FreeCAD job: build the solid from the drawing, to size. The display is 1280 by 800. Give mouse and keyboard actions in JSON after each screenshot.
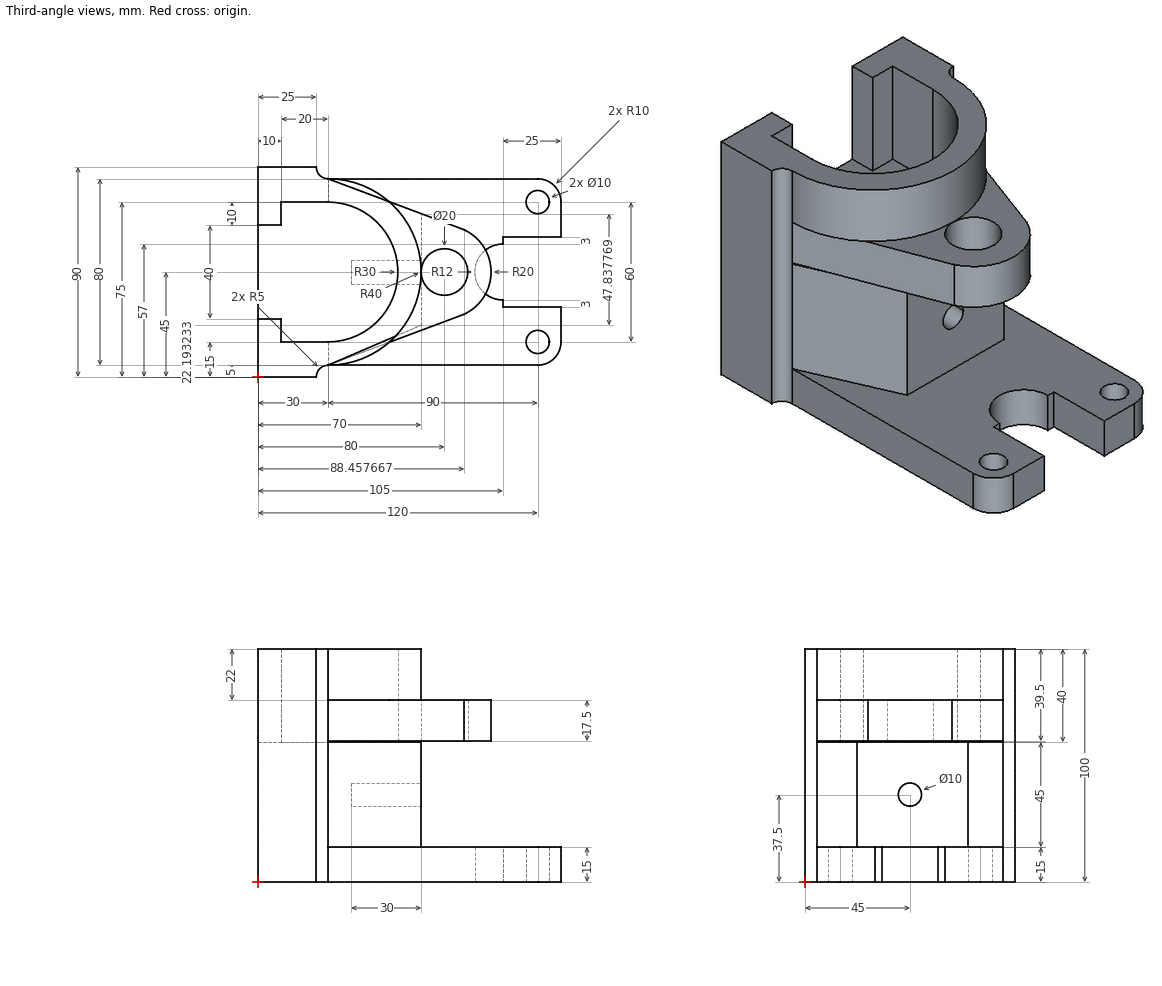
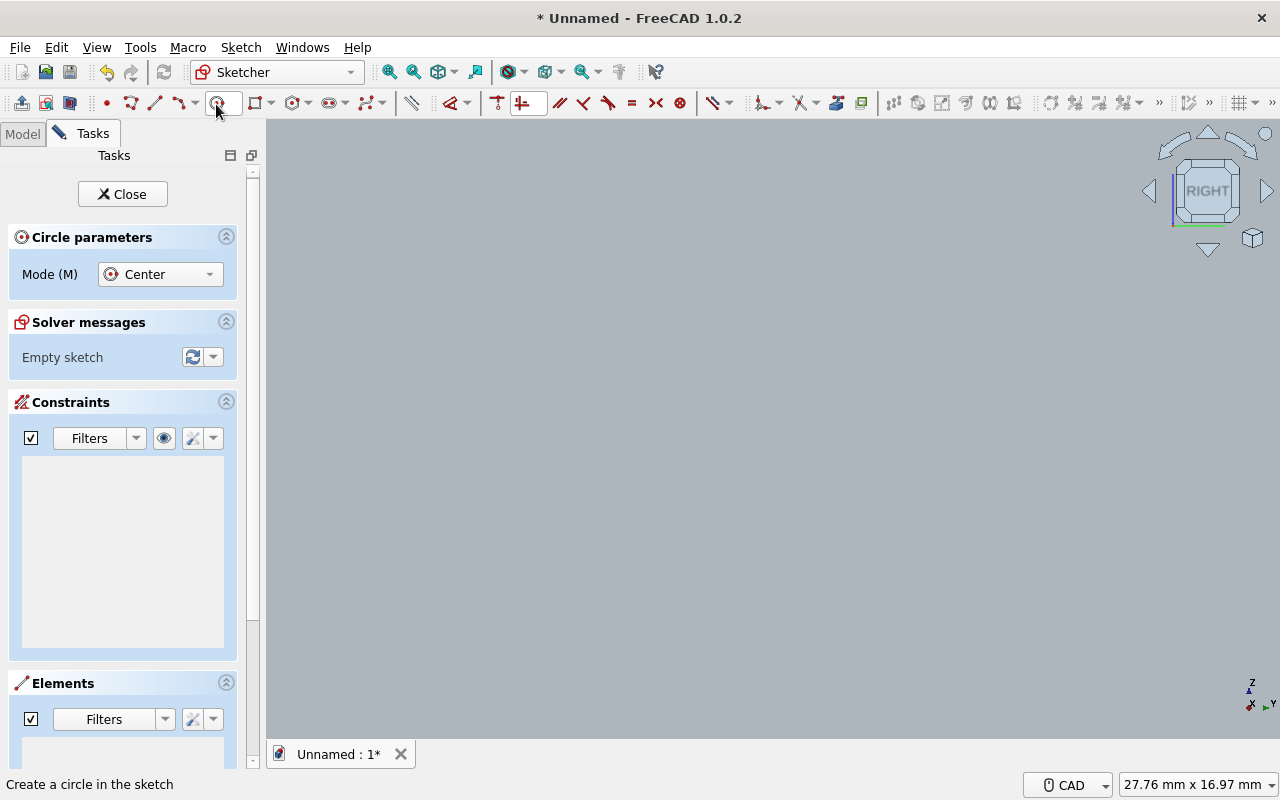
{"action": "left_click", "coordinate": [698, 419]}
{"action": "left_click", "coordinate": [827, 290]}
{"action": "key", "text": "Escape"}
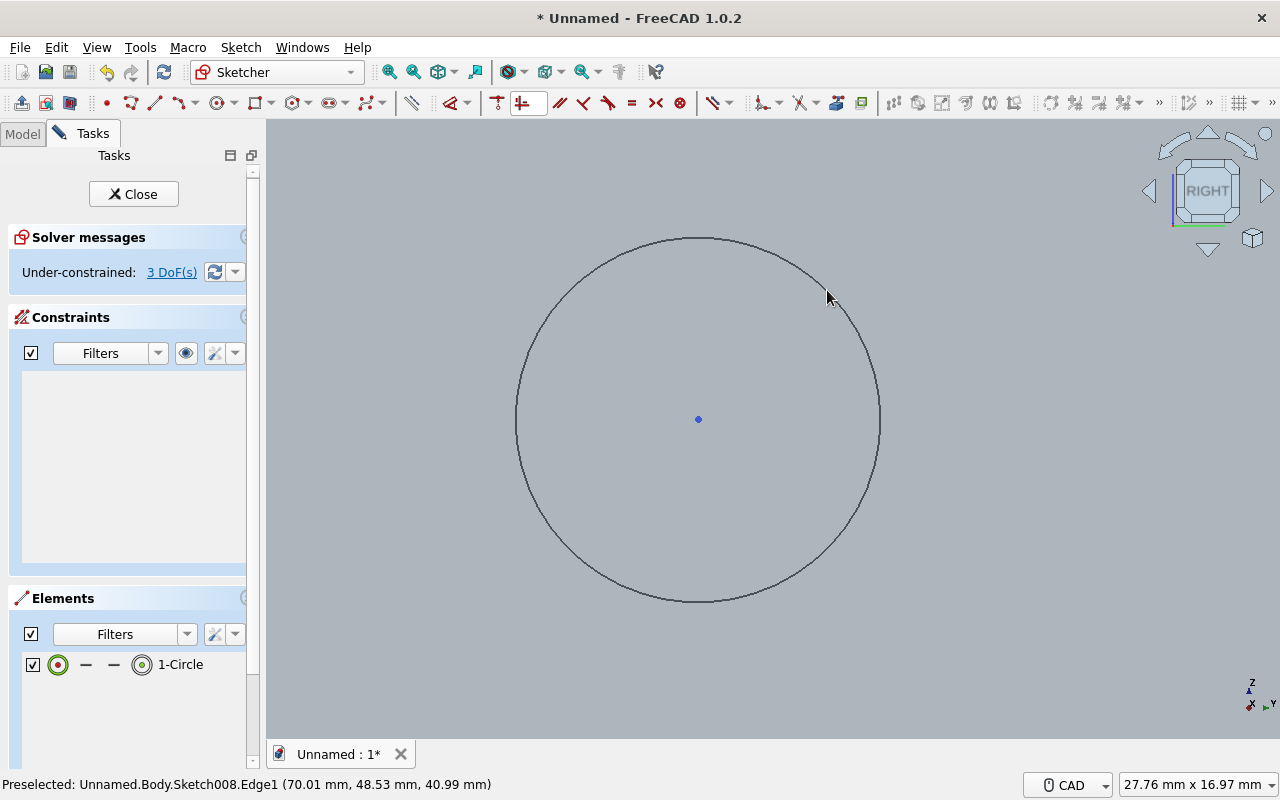
{"action": "left_click", "coordinate": [450, 104]}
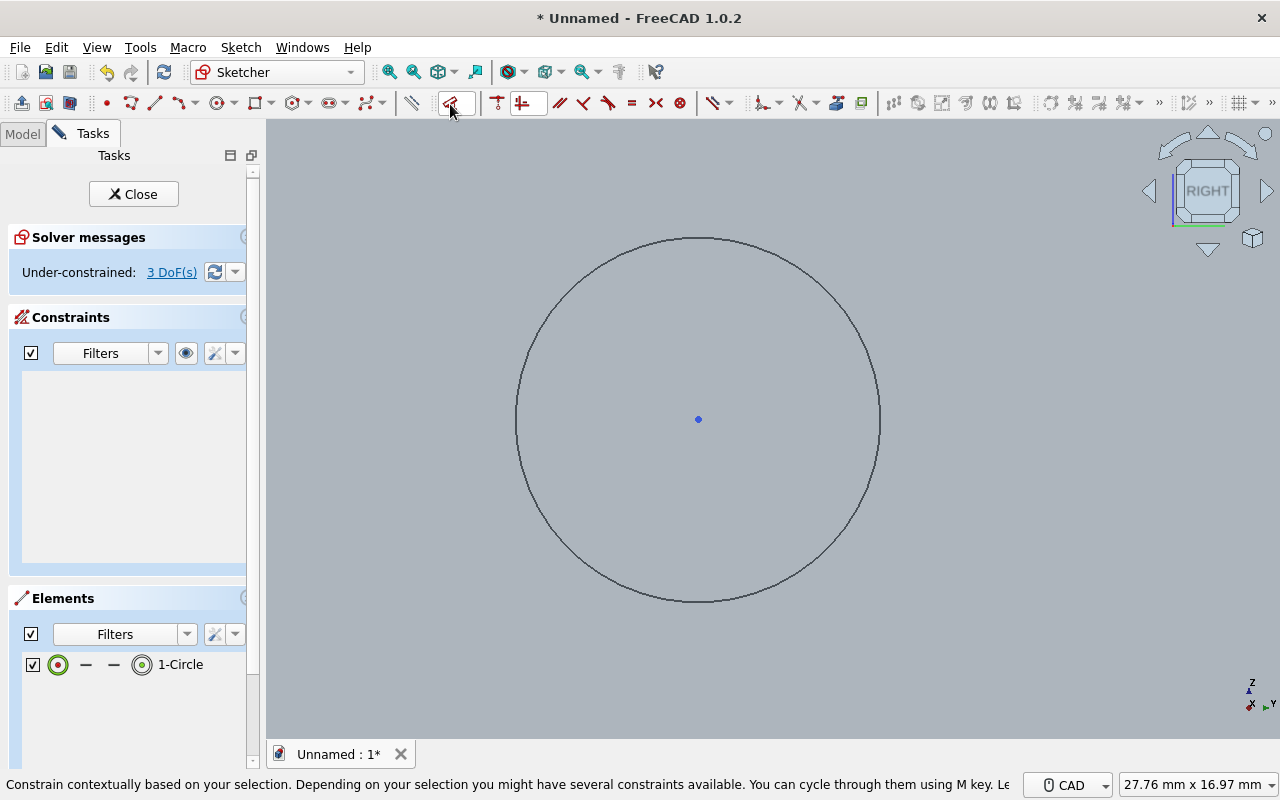
{"action": "left_click", "coordinate": [827, 291]}
{"action": "left_click", "coordinate": [850, 268]}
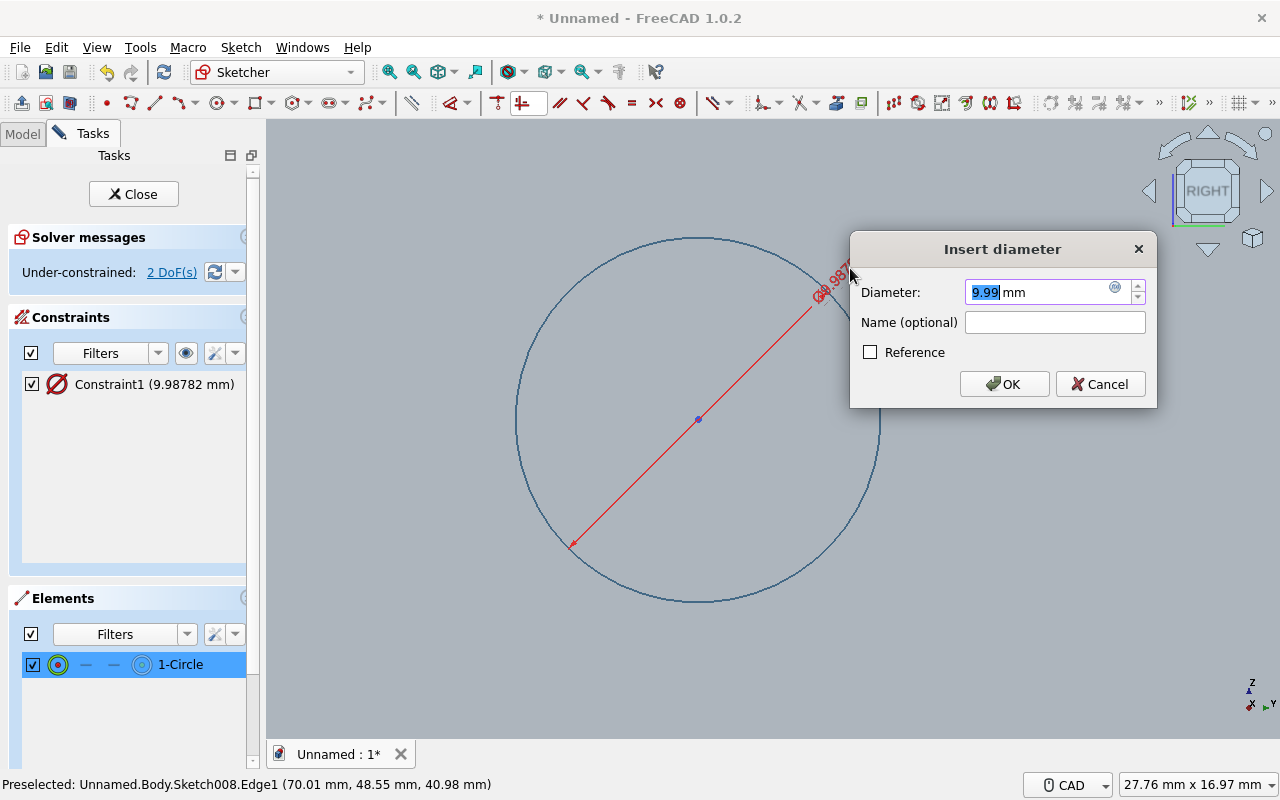
{"action": "type", "text": "10"}
{"action": "key", "text": "Return"}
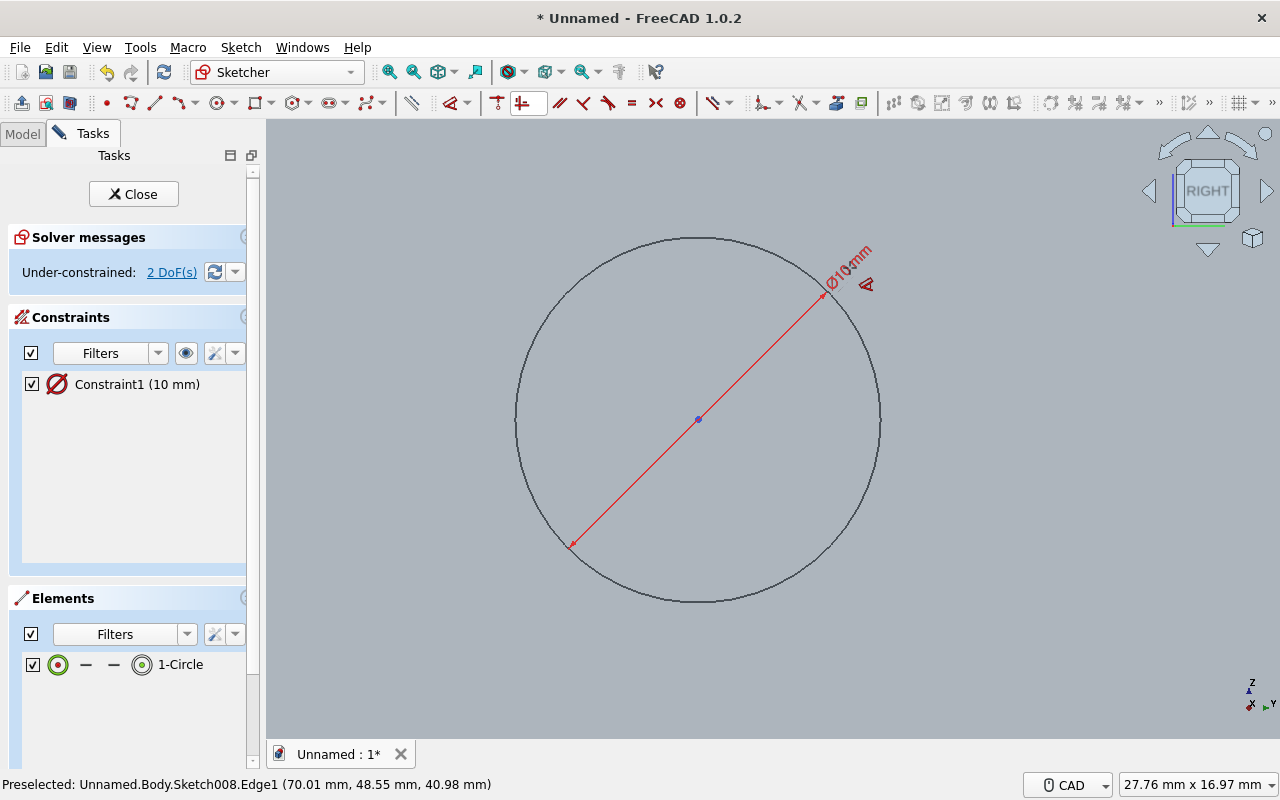
{"action": "left_click", "coordinate": [698, 420]}
{"action": "left_click", "coordinate": [496, 386]}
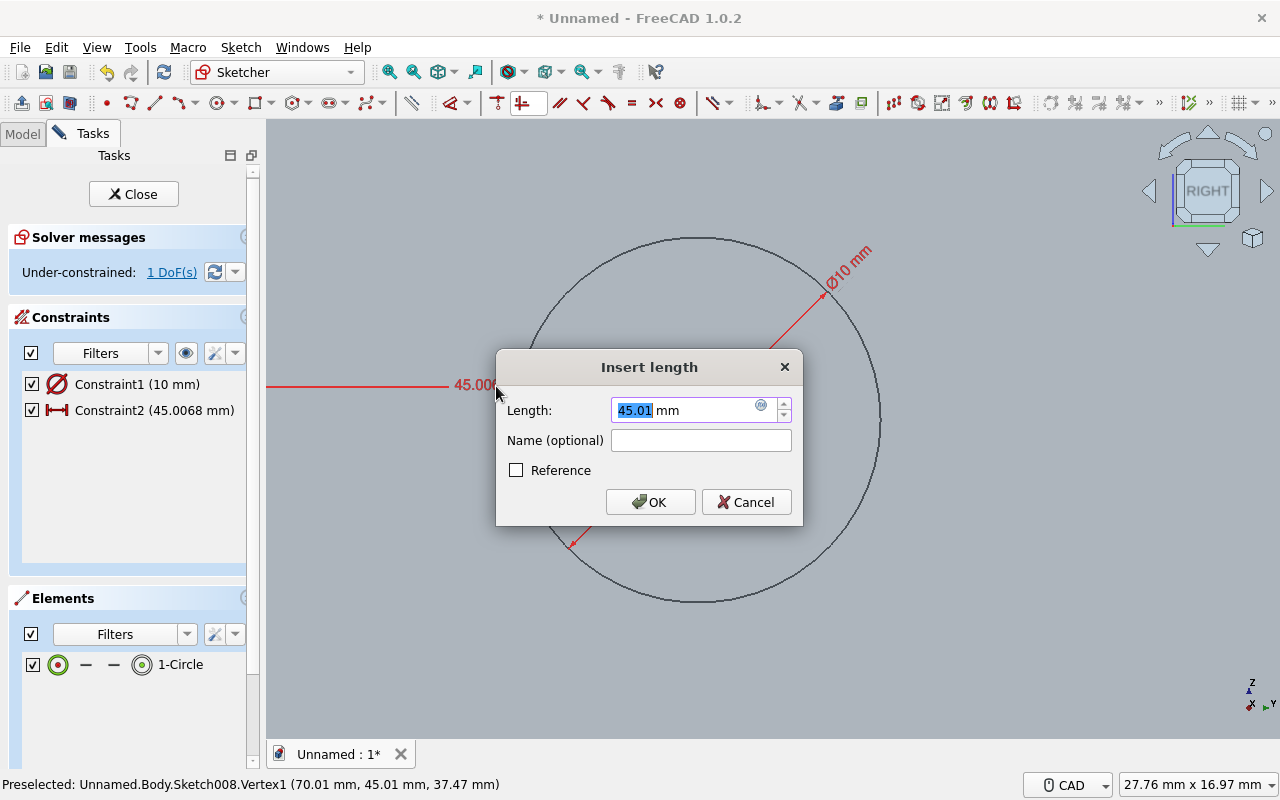
{"action": "type", "text": "45"}
{"action": "key", "text": "Return"}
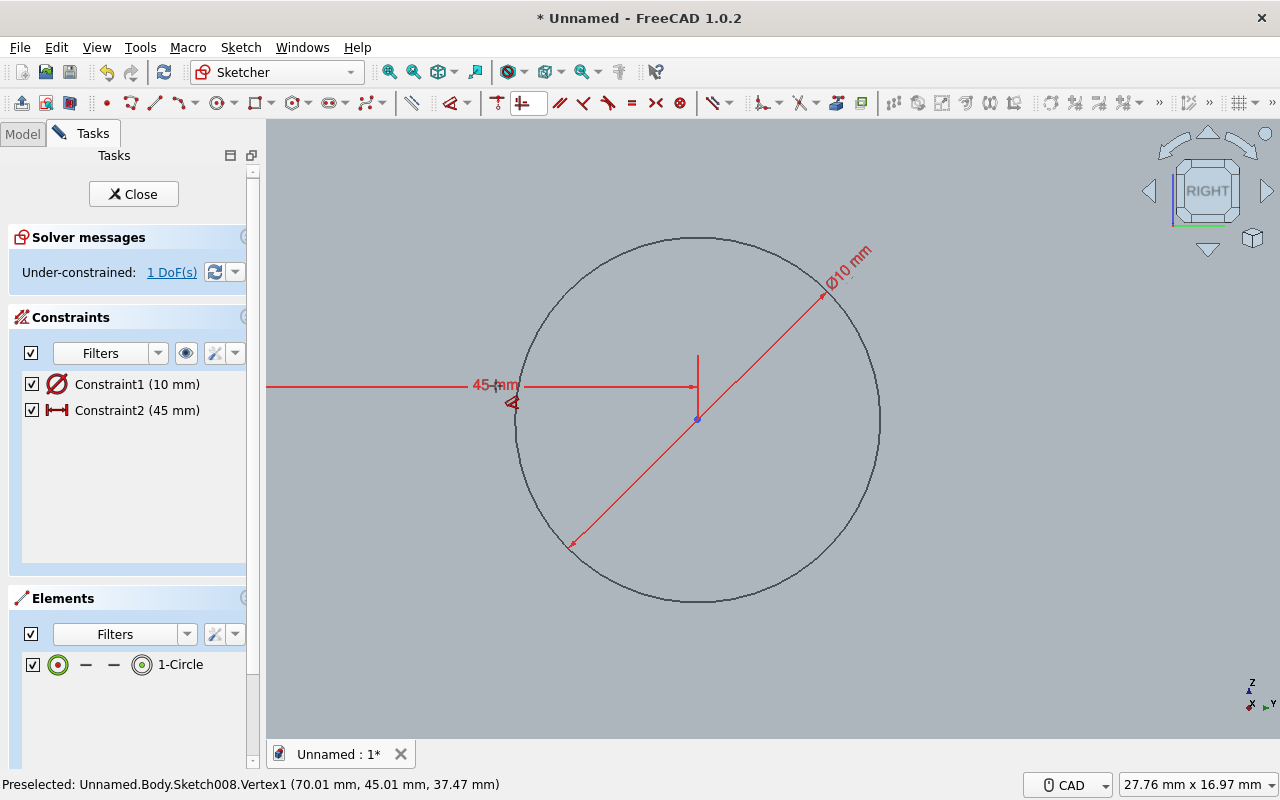
{"action": "left_click", "coordinate": [698, 420]}
{"action": "left_click", "coordinate": [732, 566]}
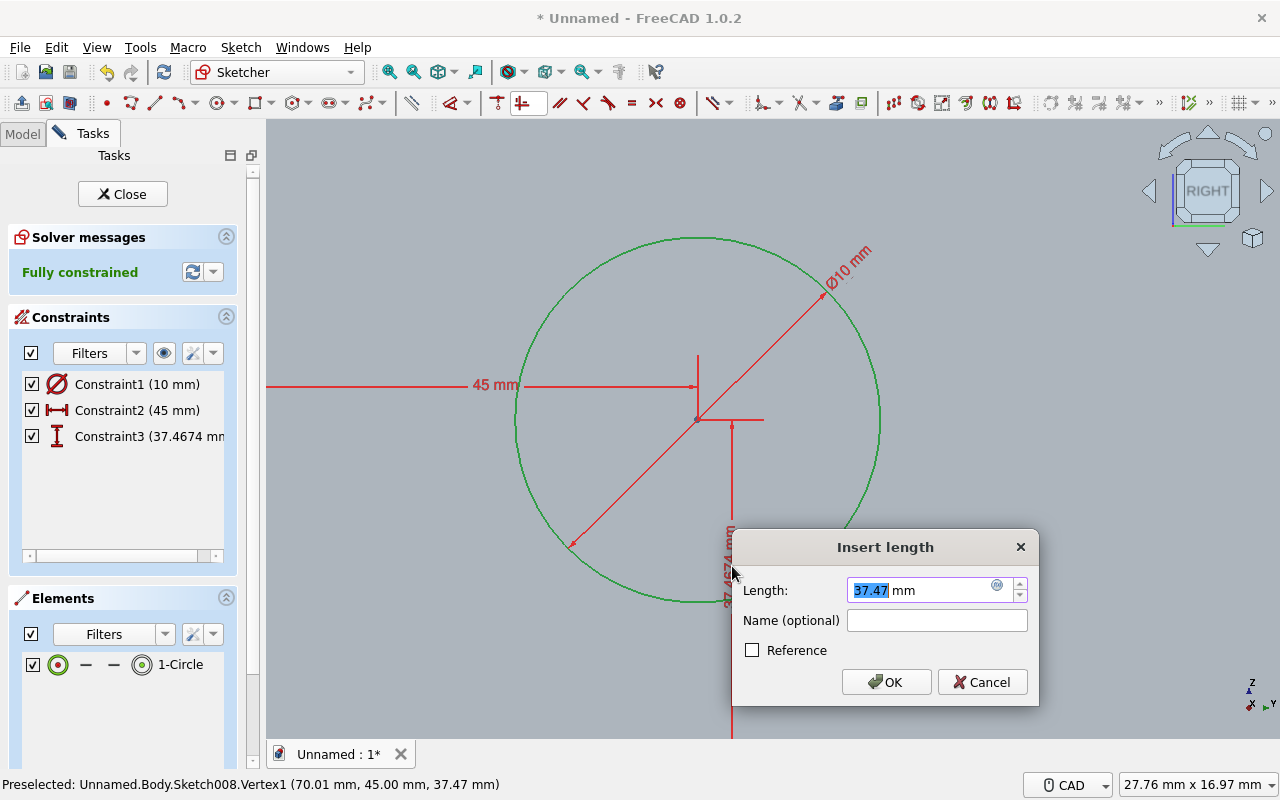
{"action": "type", "text": "37.5"}
{"action": "key", "text": "Return"}
{"action": "key", "text": "Escape"}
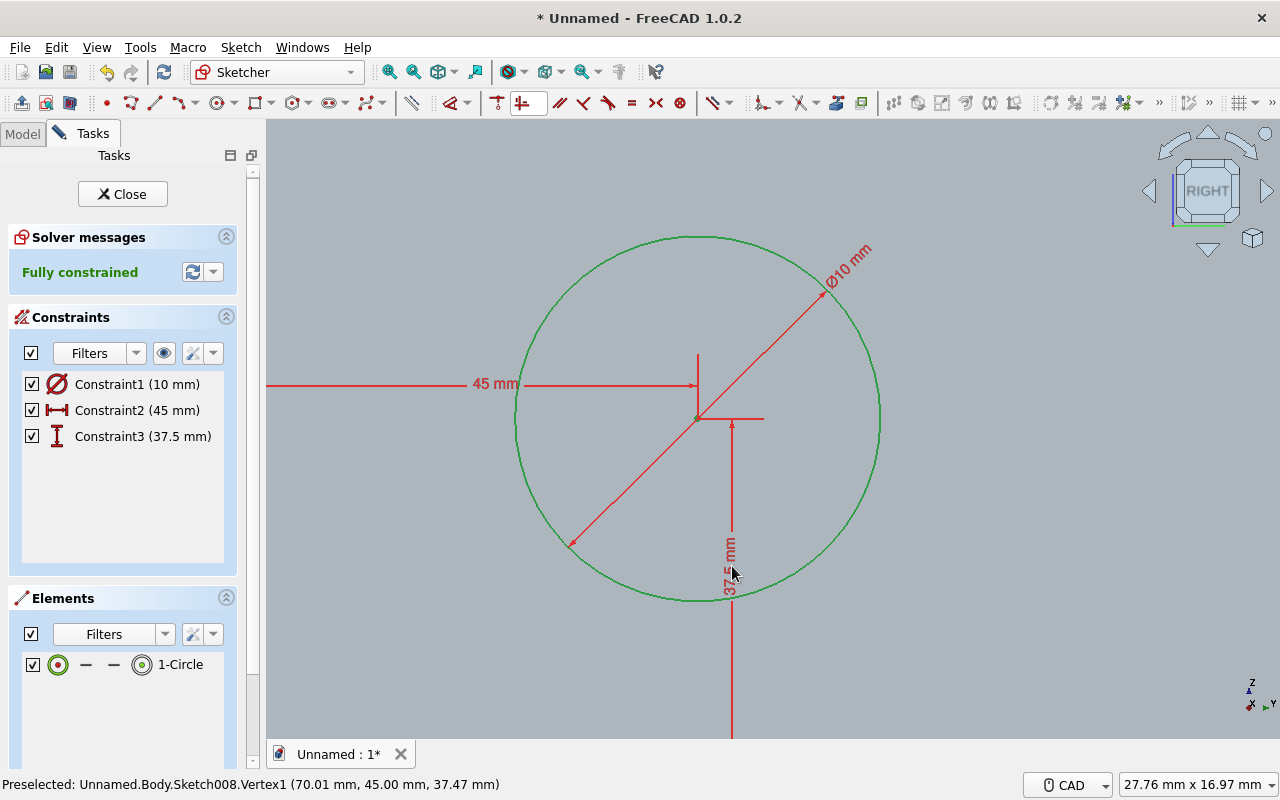
{"action": "left_click", "coordinate": [123, 194]}